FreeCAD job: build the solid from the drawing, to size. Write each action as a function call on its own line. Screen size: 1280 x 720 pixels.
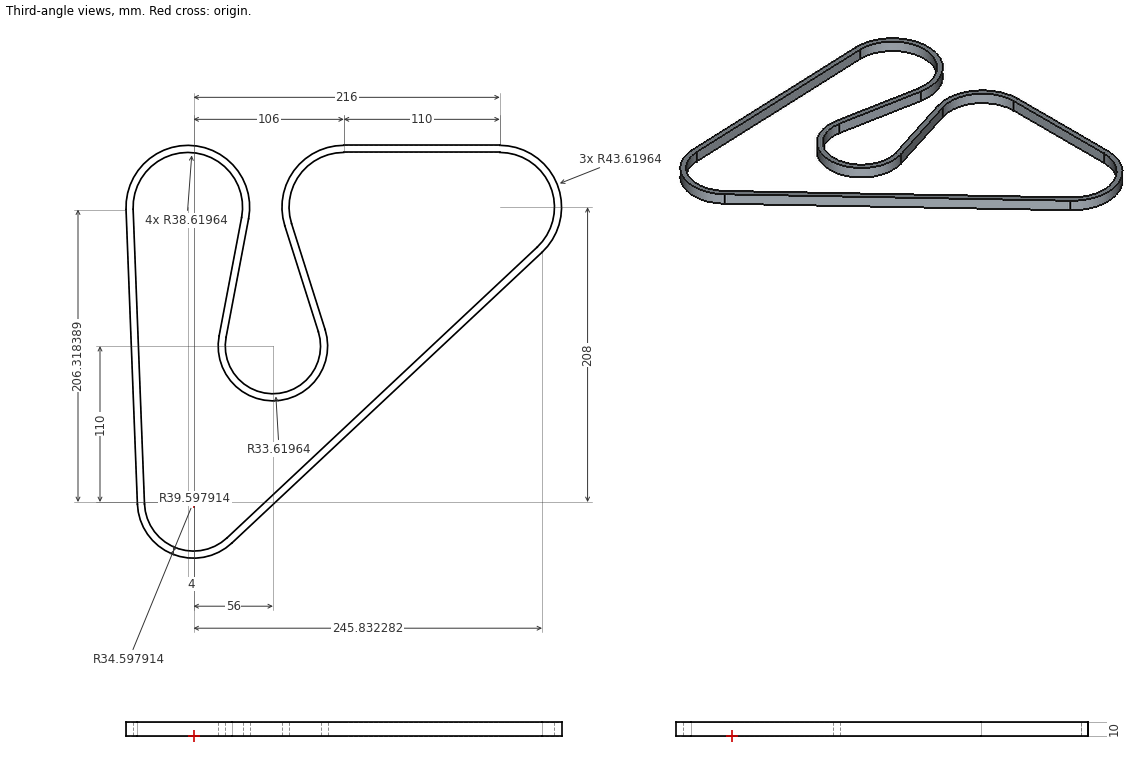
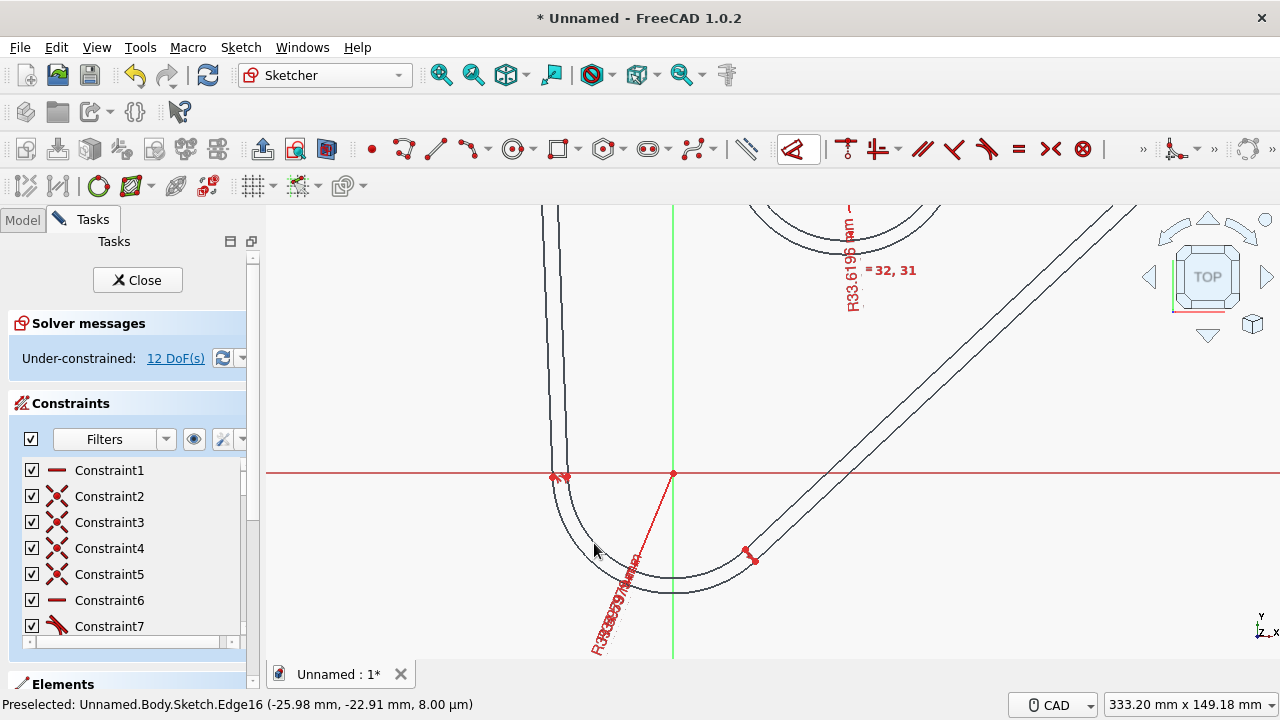
scroll(581, 555, down, 6)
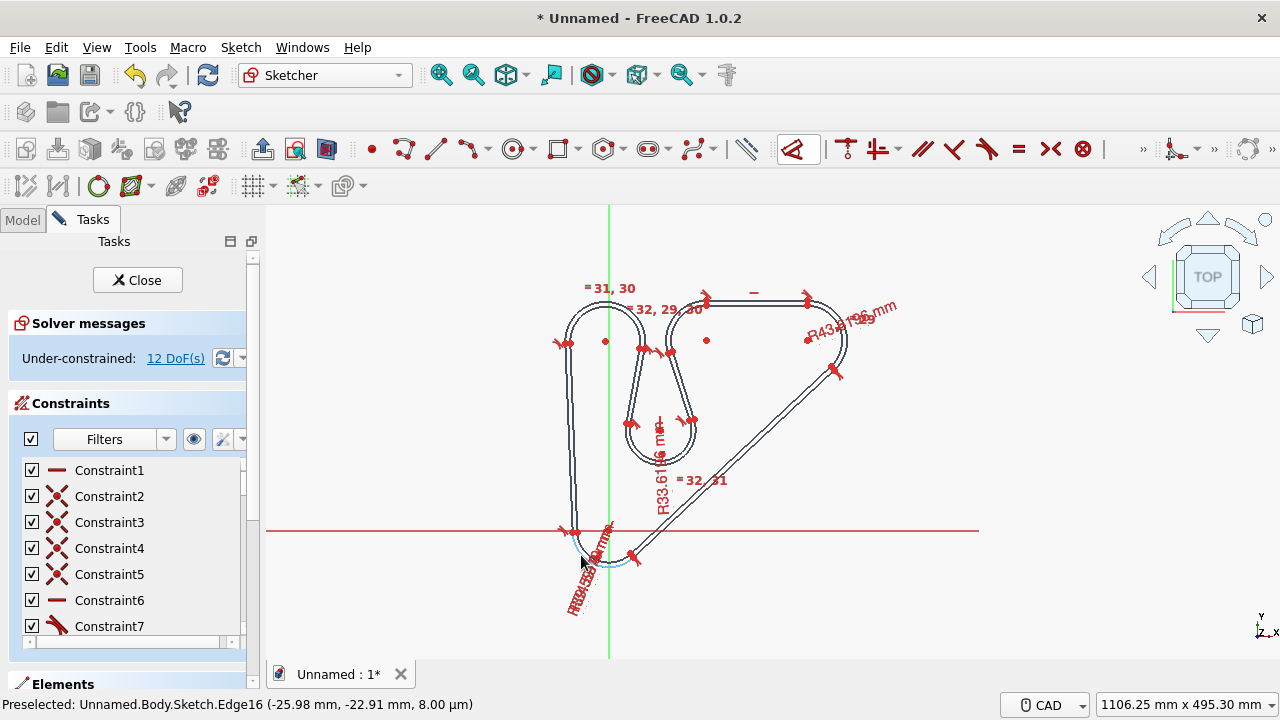
scroll(629, 316, up, 6)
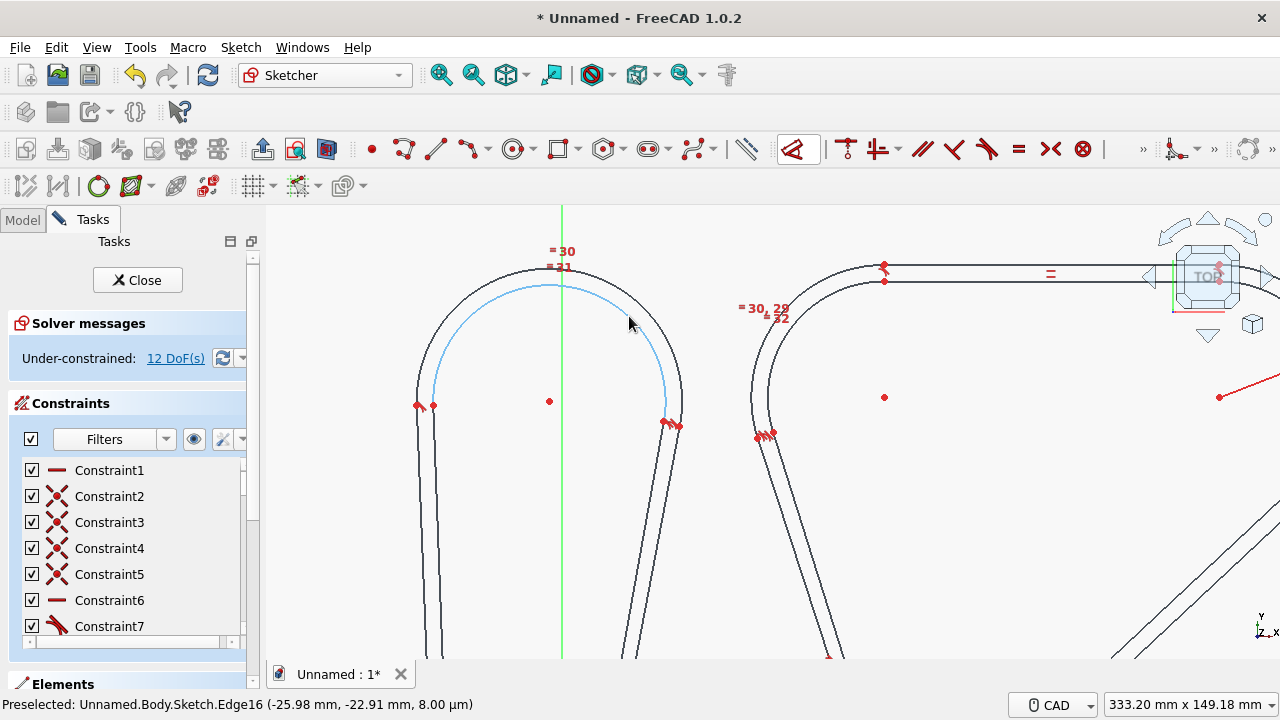
click(628, 316)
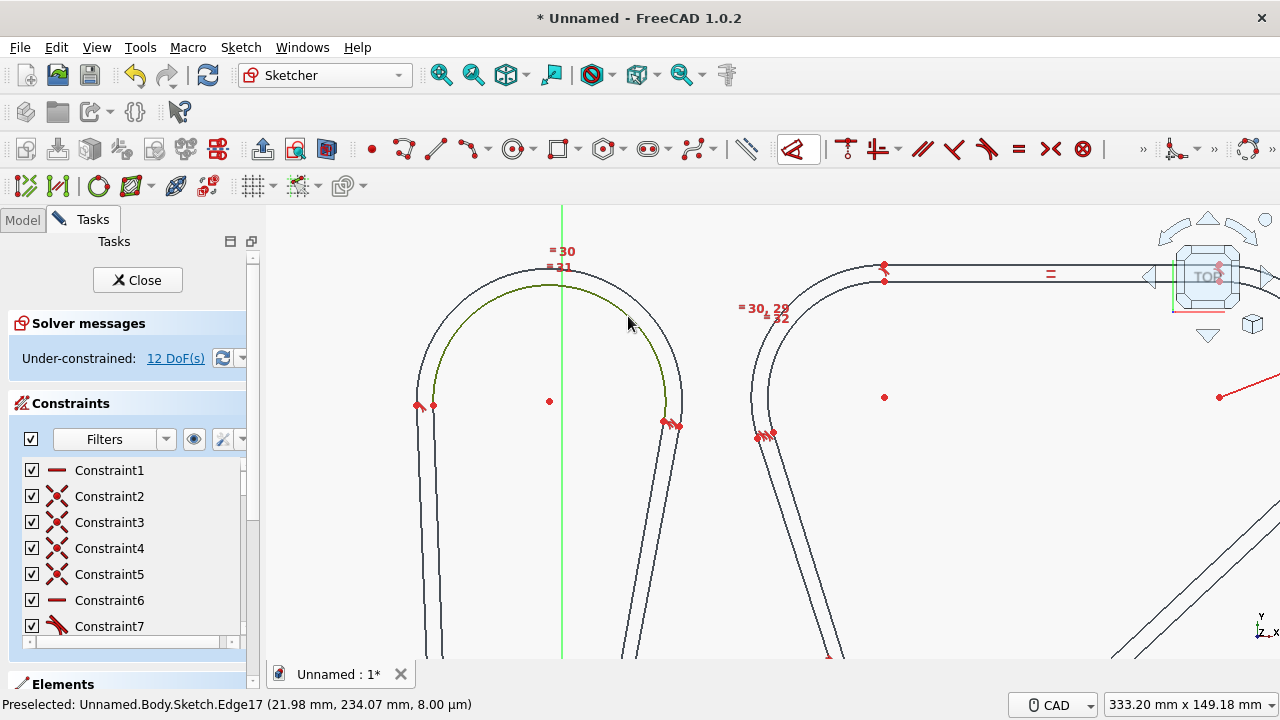
click(814, 150)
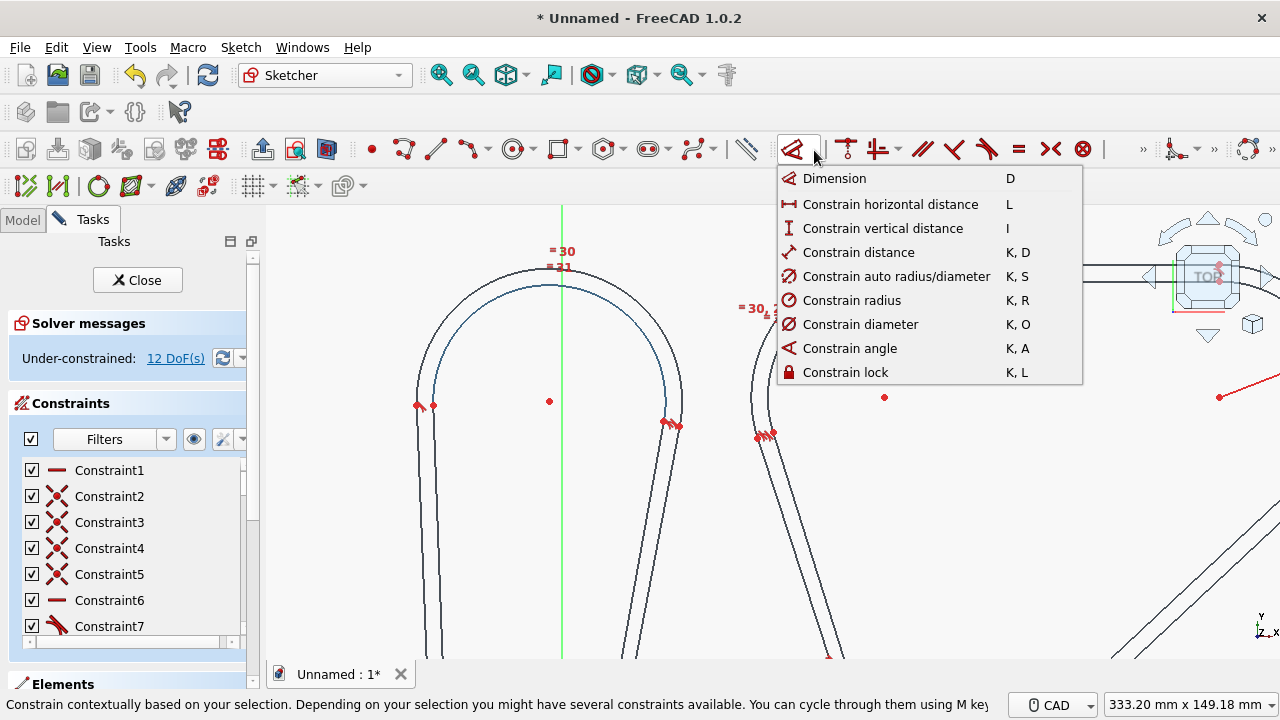
click(930, 300)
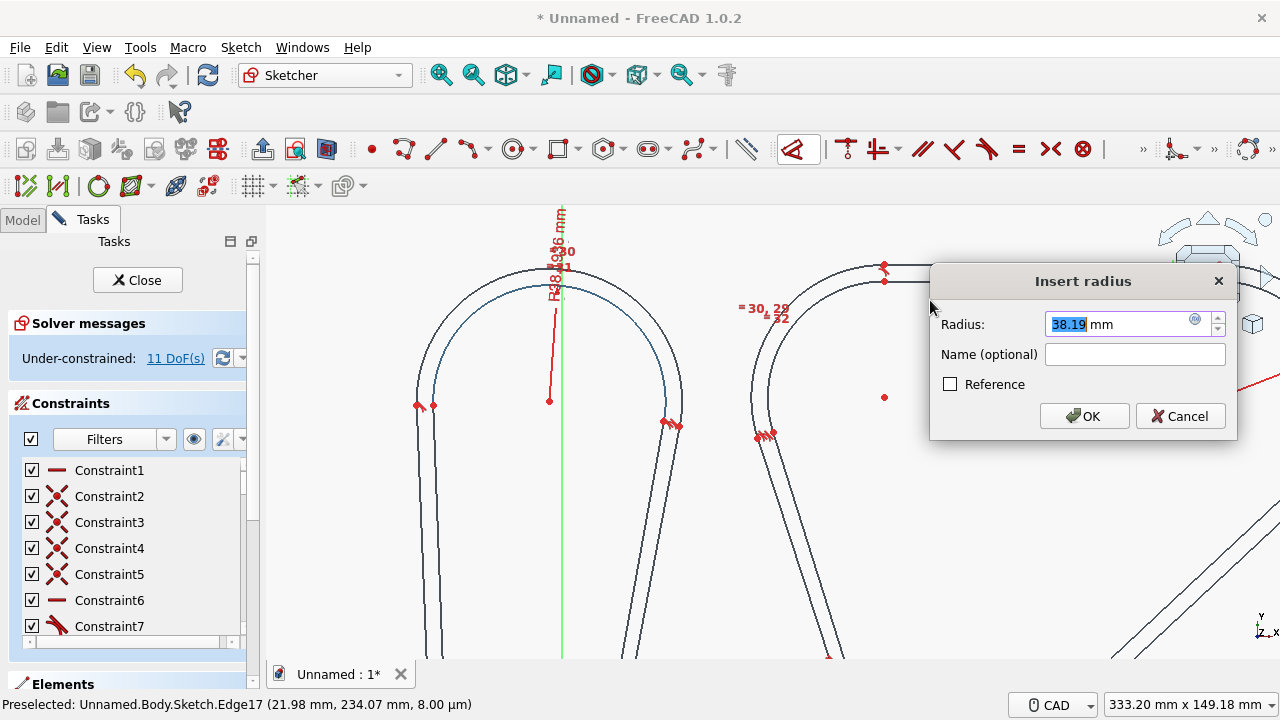
text(38.61964)
key(Return)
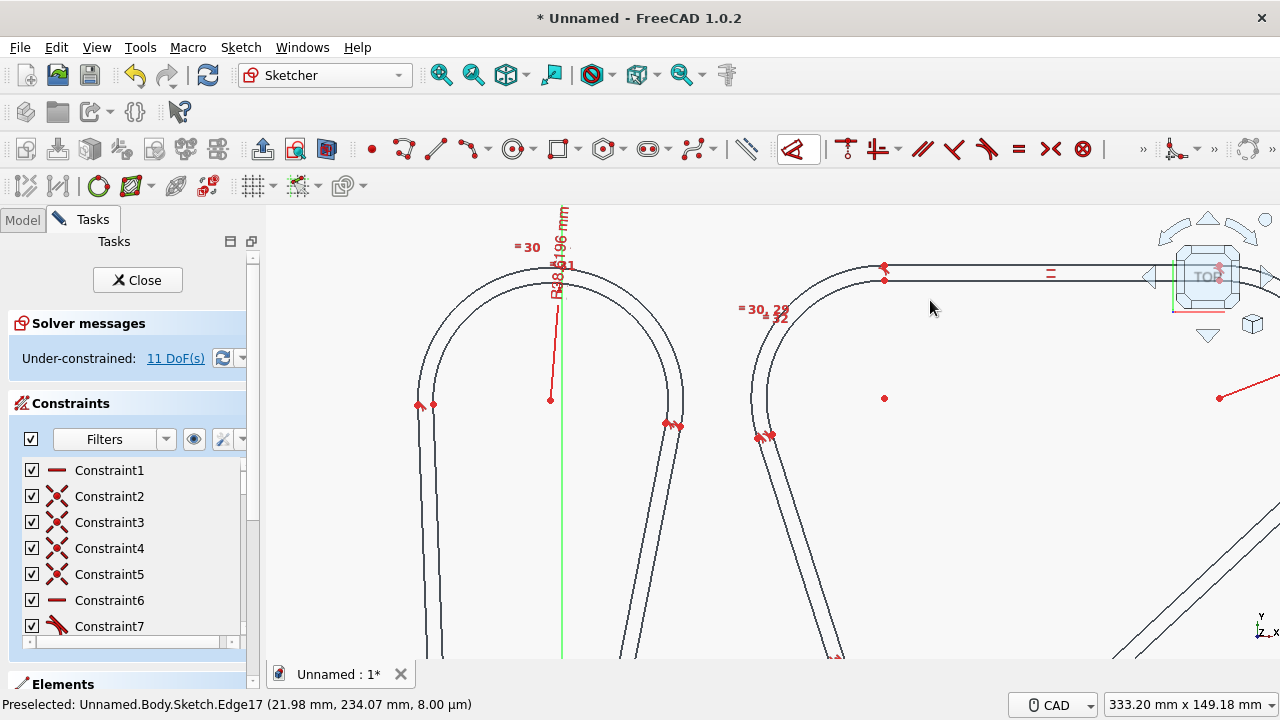
scroll(551, 401, up, 6)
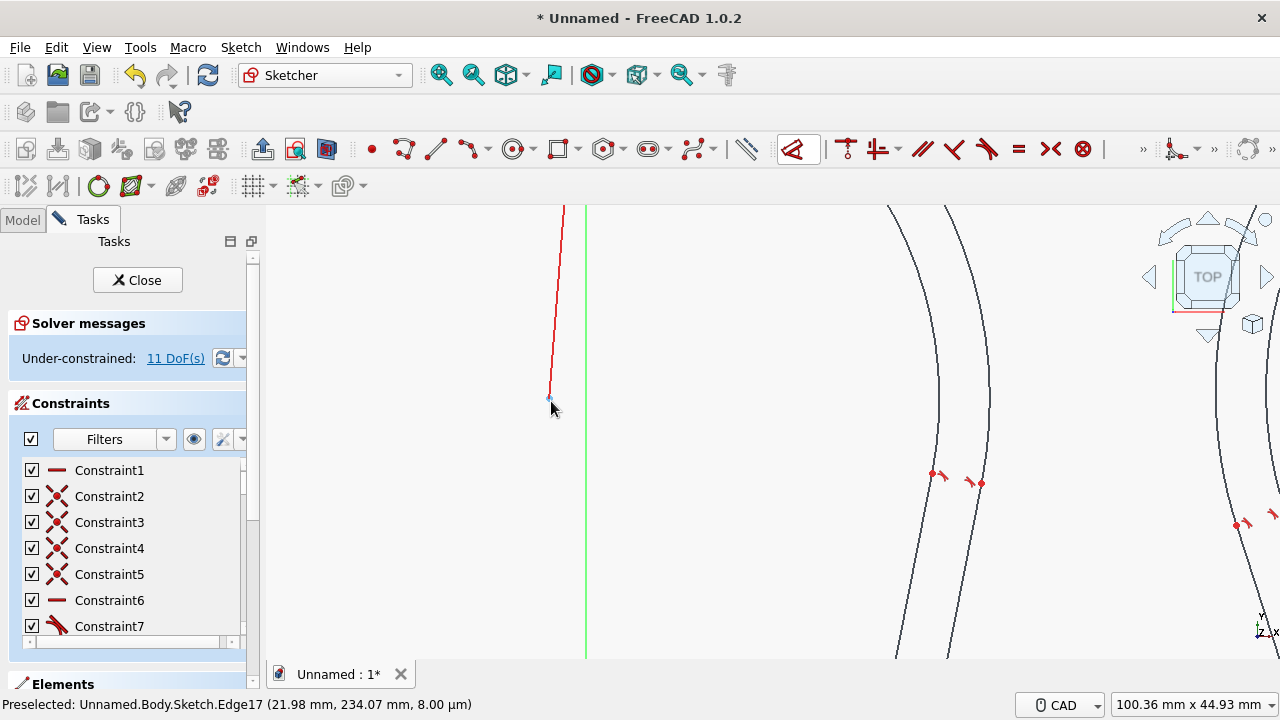
click(549, 399)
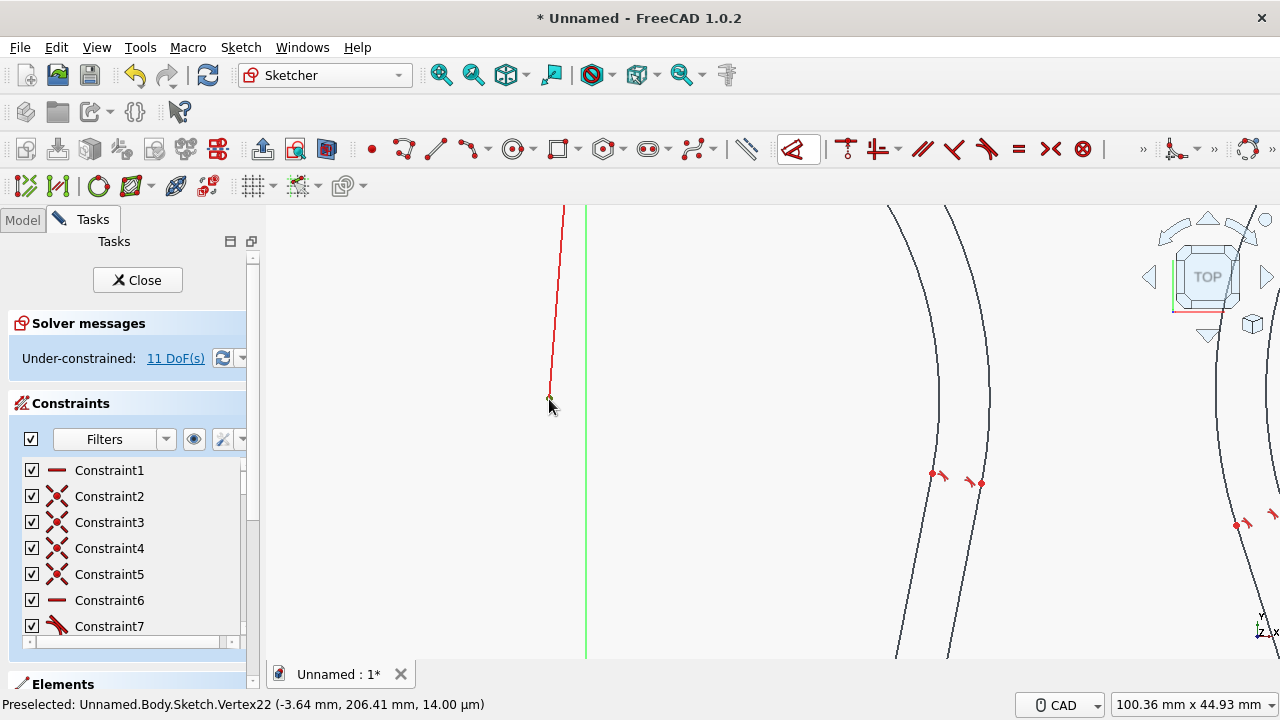
key(l)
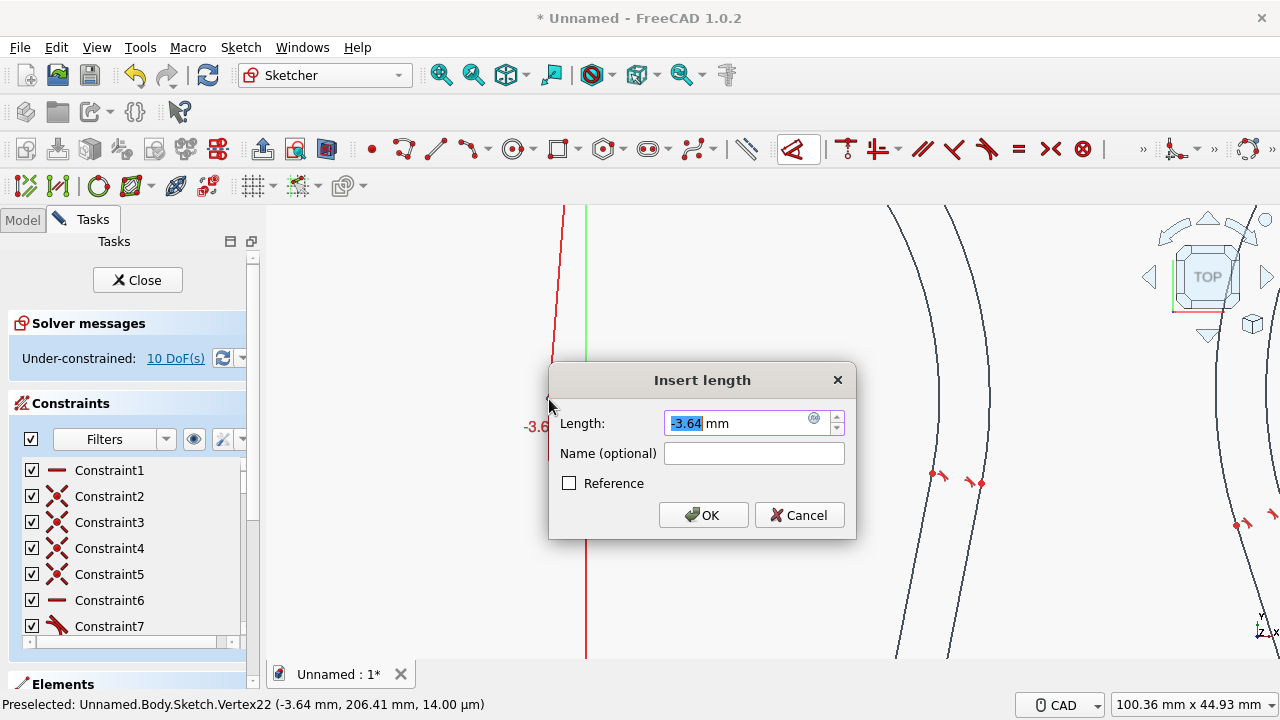
text(-4)
key(Return)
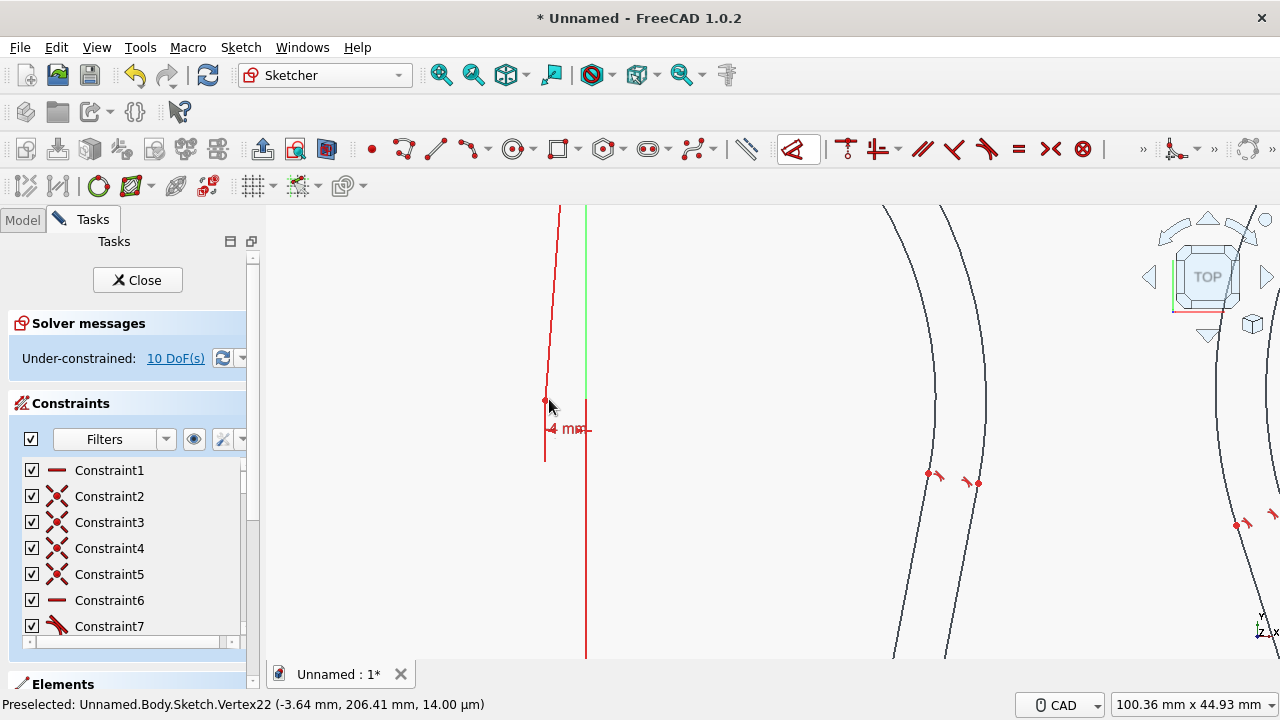
scroll(611, 336, down, 12)